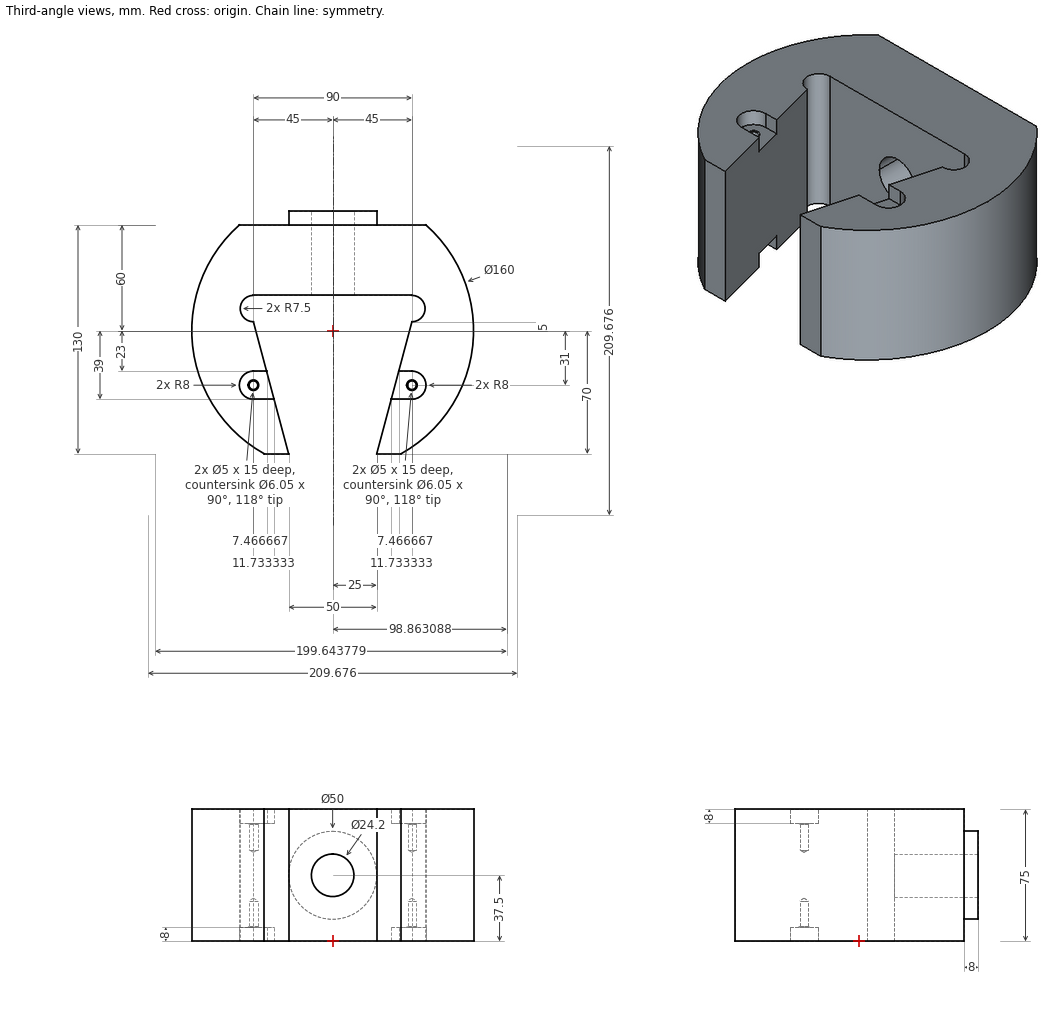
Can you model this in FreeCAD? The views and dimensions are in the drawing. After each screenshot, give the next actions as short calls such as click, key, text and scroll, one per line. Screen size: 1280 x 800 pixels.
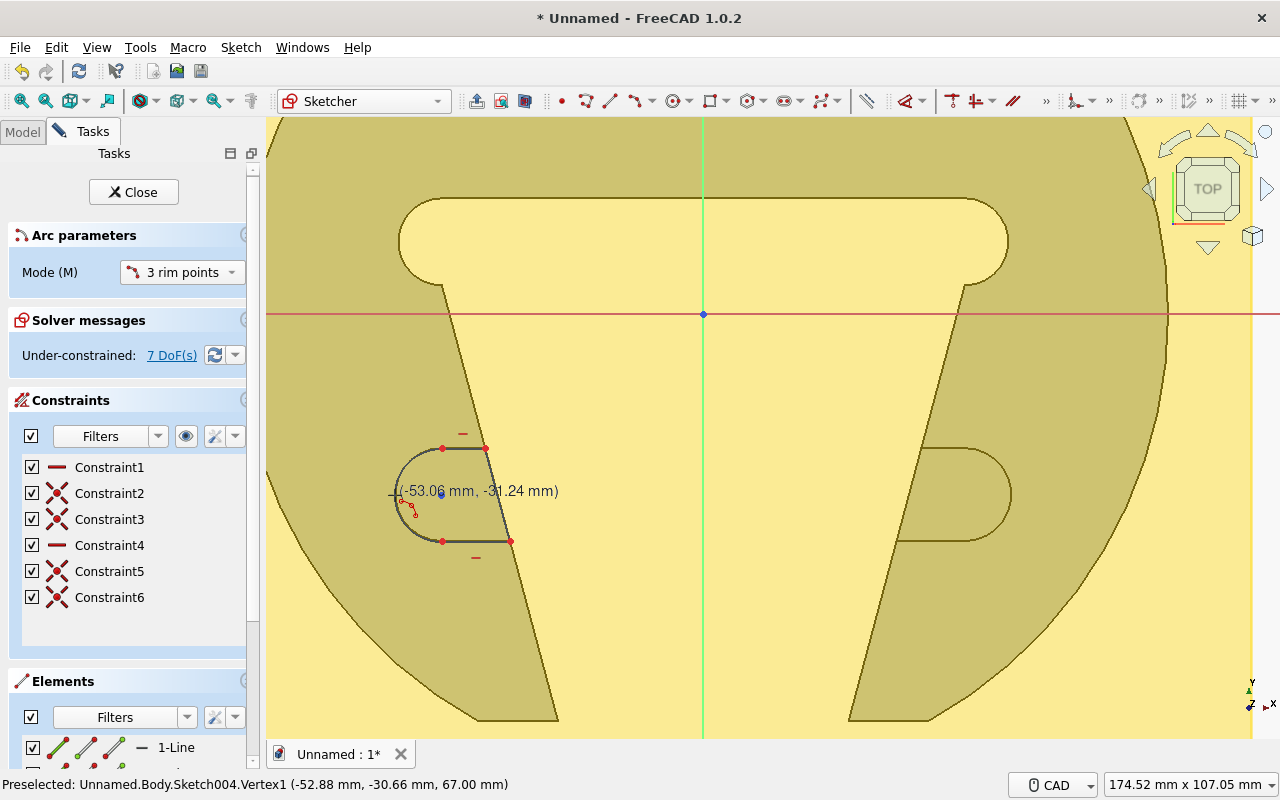
key(g)
key(m)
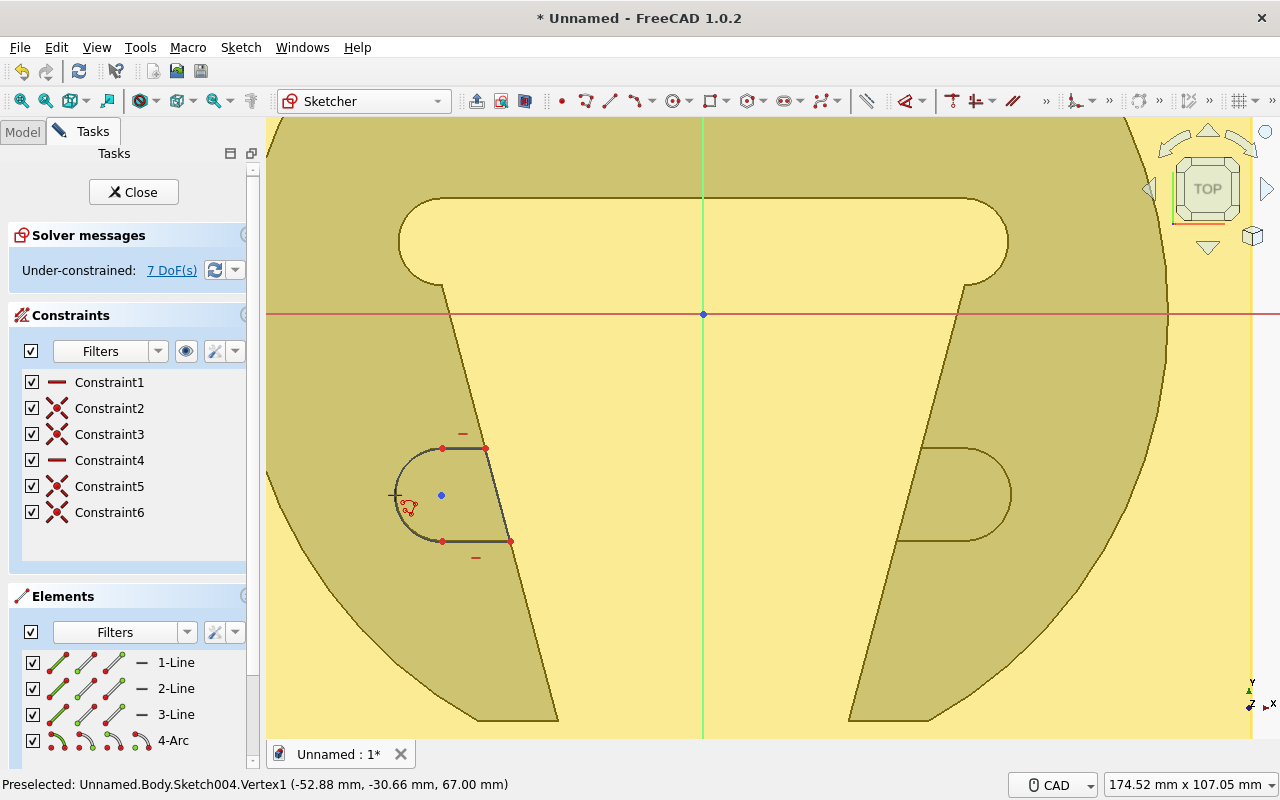
click(965, 541)
click(897, 541)
click(921, 448)
click(965, 448)
right_click(965, 448)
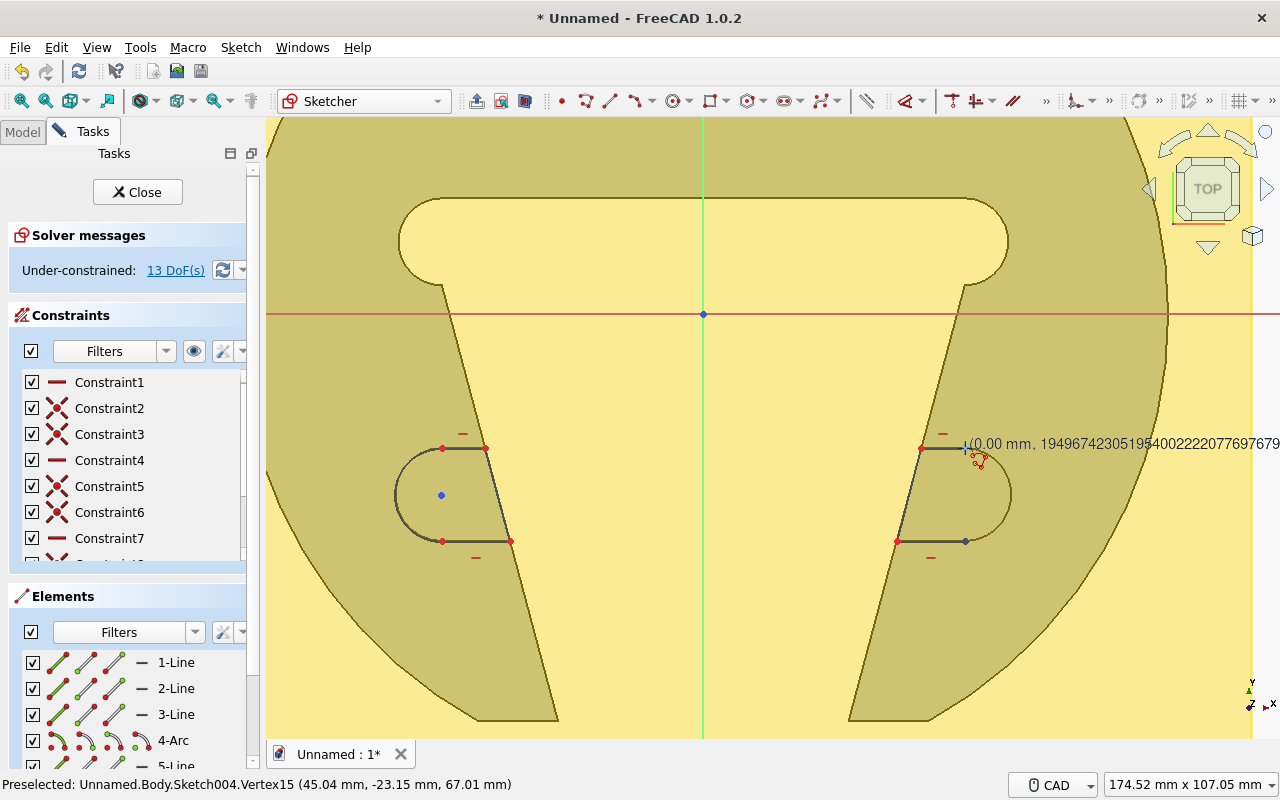
key(g)
key(3)
key(a)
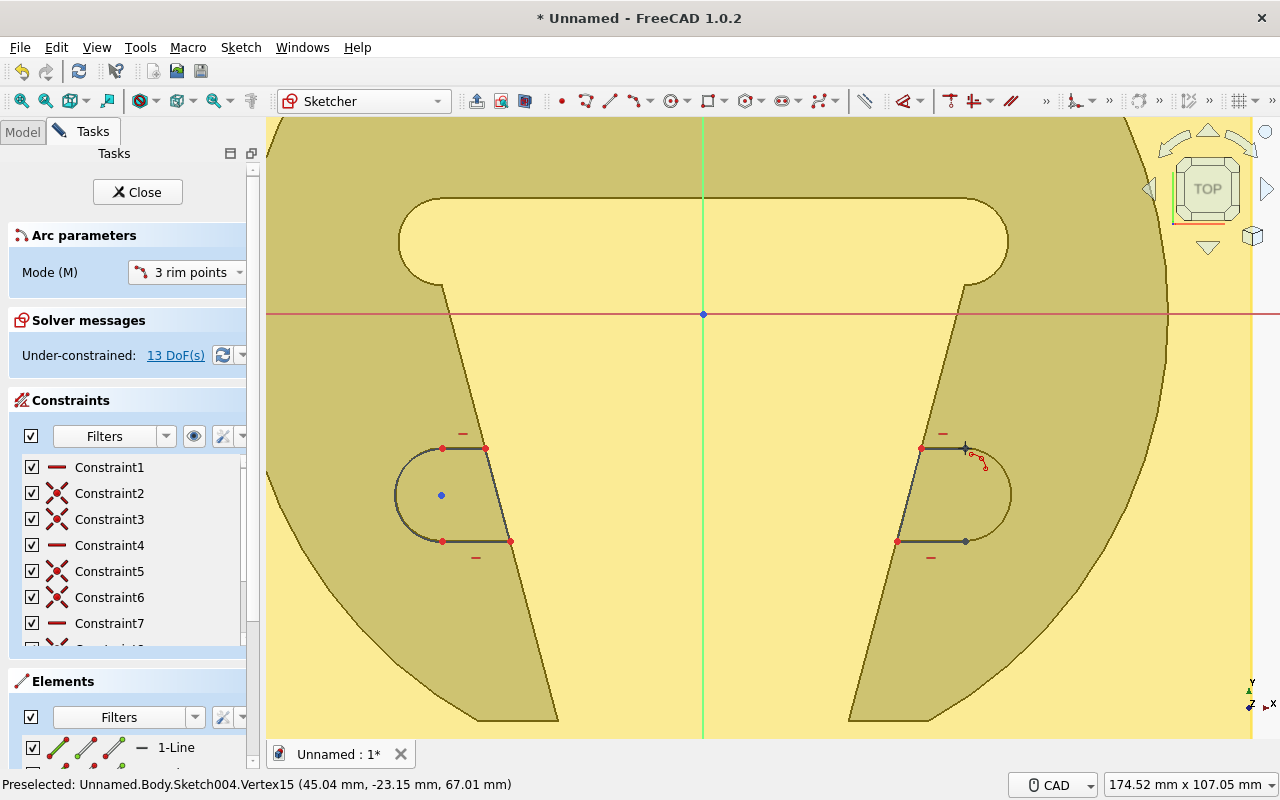
click(965, 449)
click(965, 542)
click(1011, 495)
key(Escape)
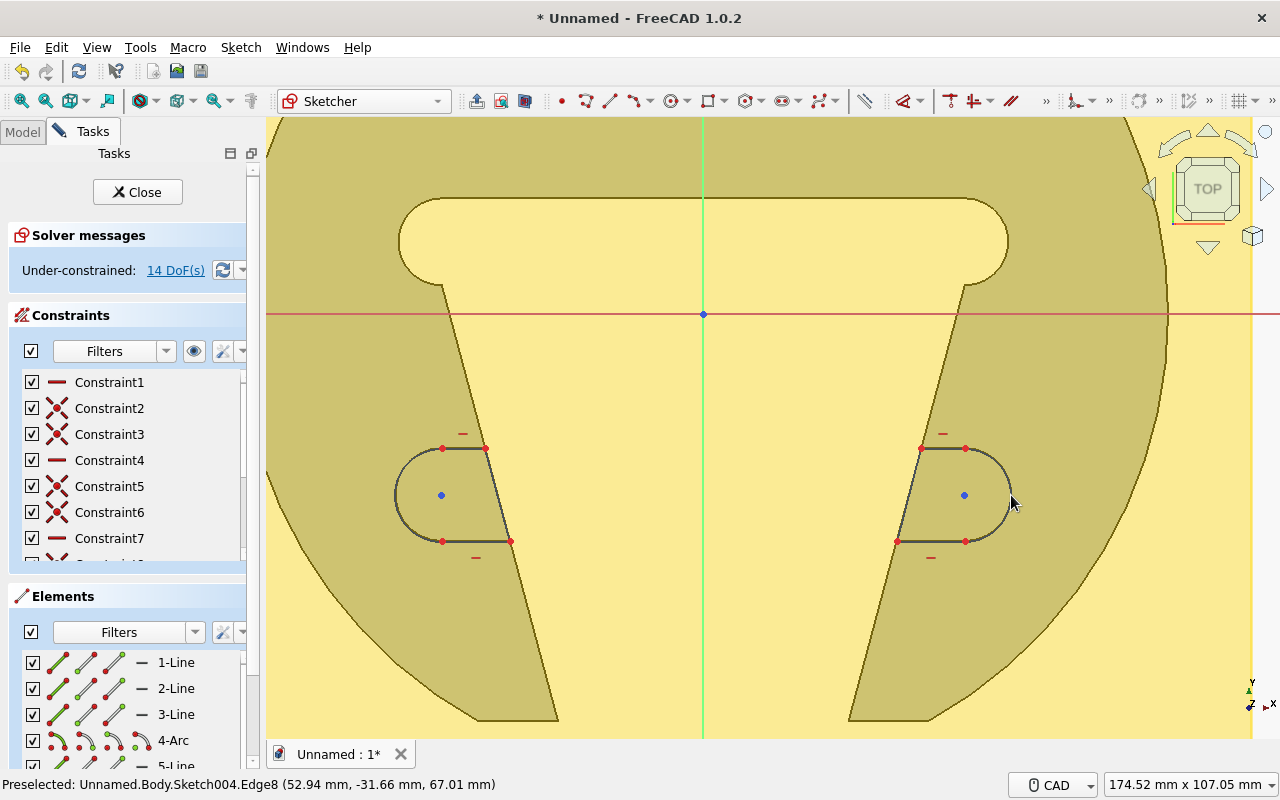
click(455, 449)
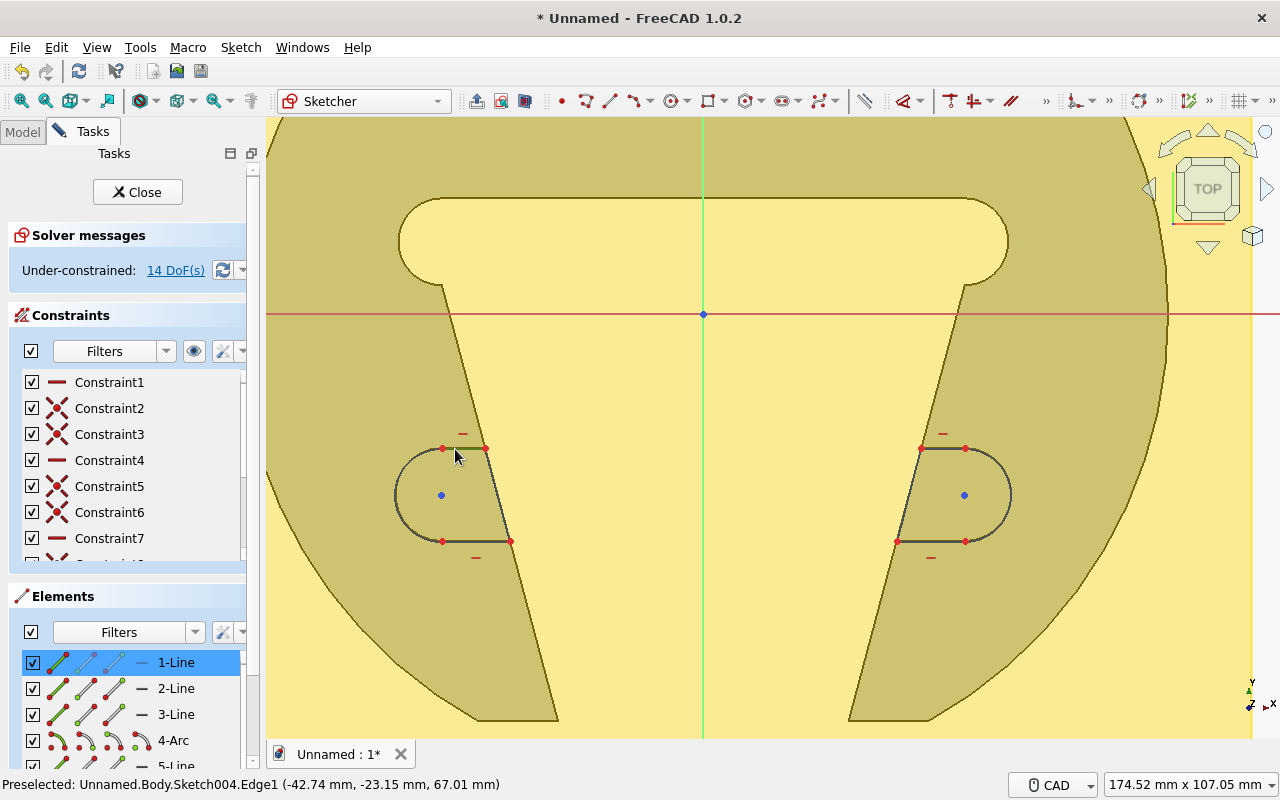
click(404, 468)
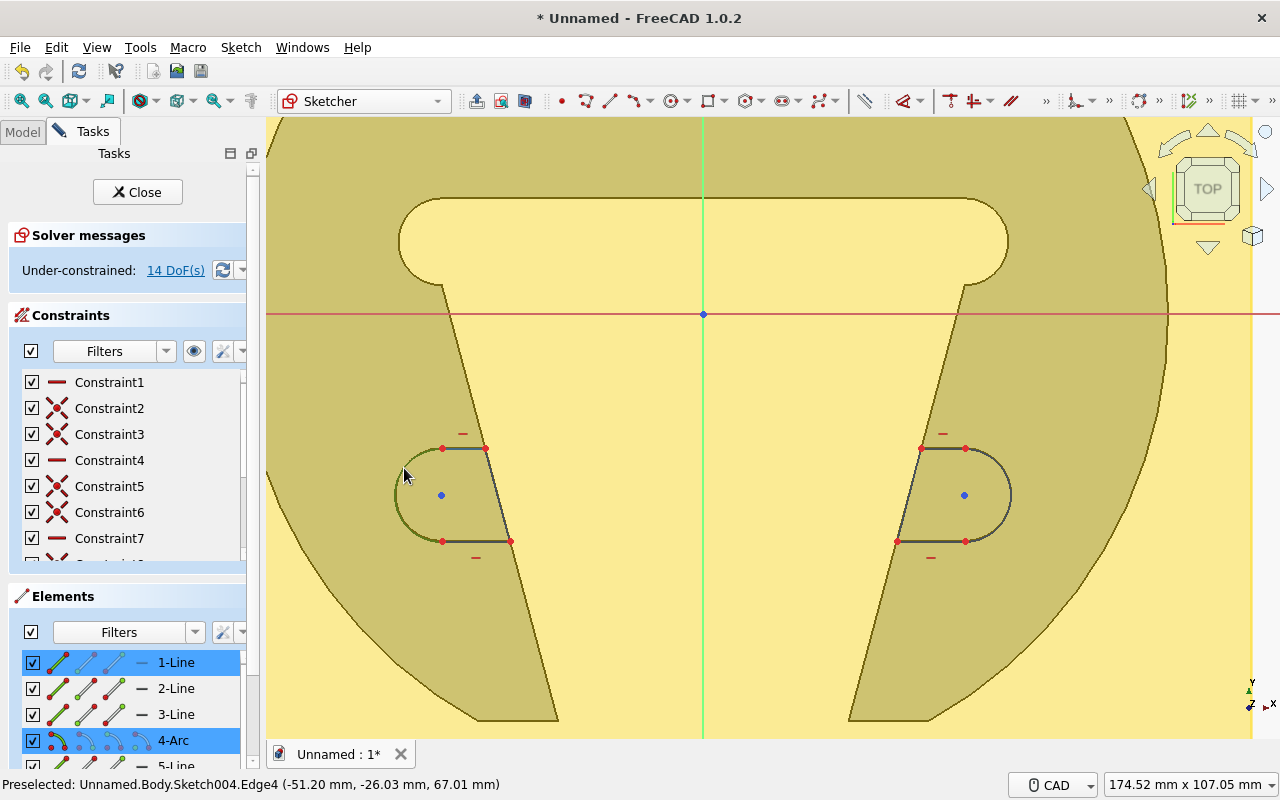
key(t)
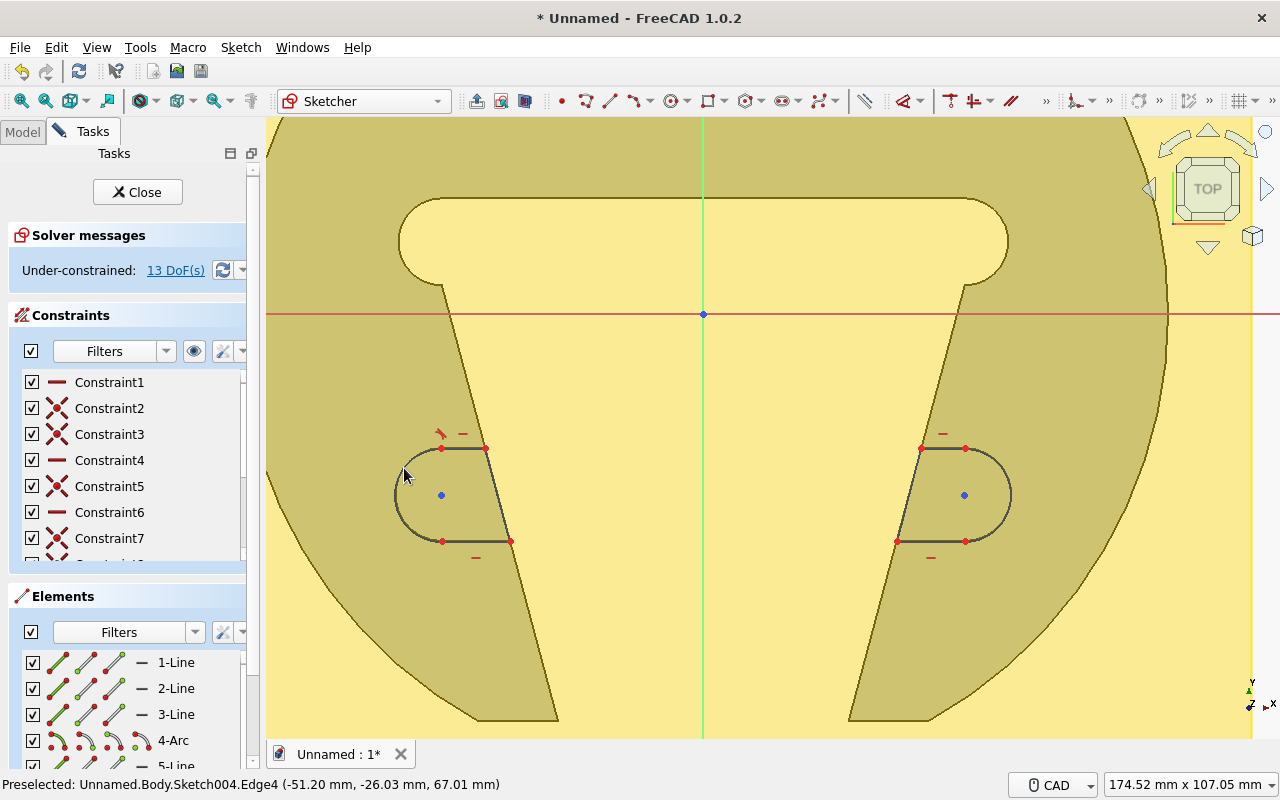
click(490, 542)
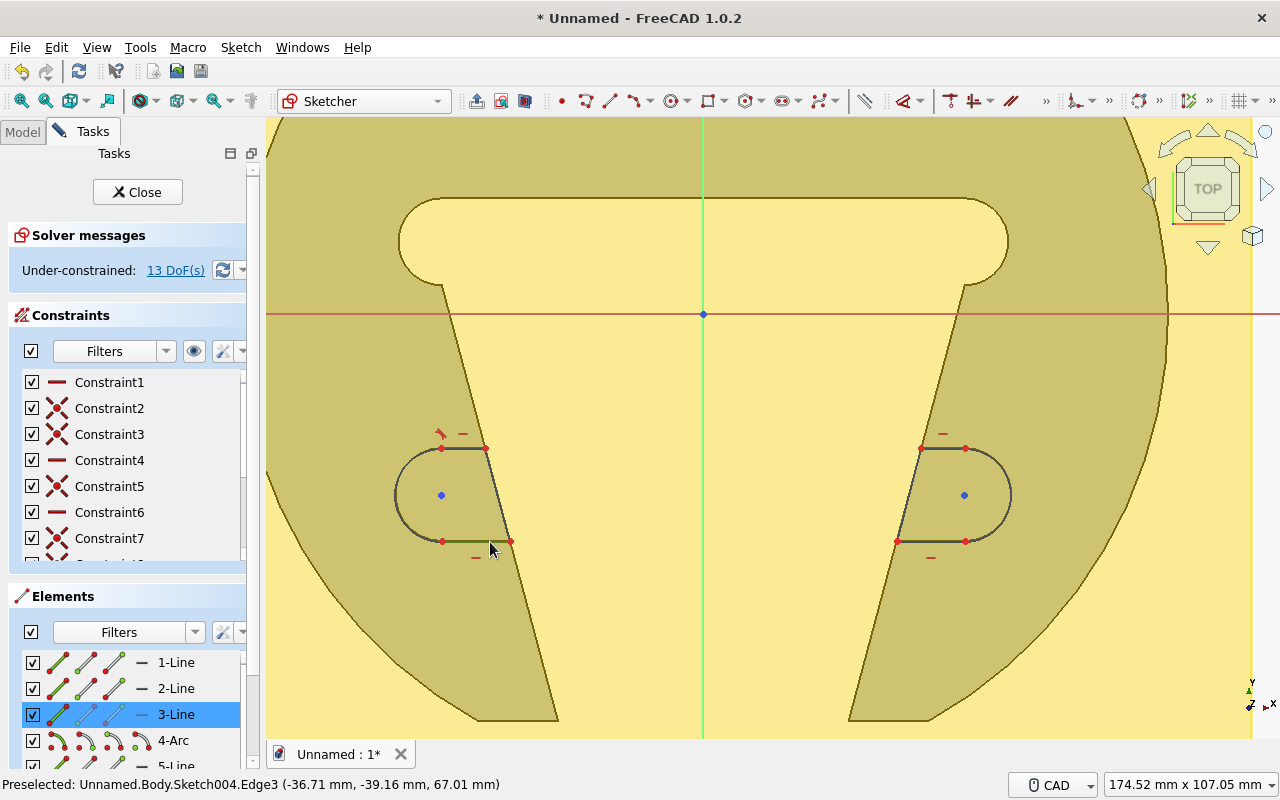
click(404, 468)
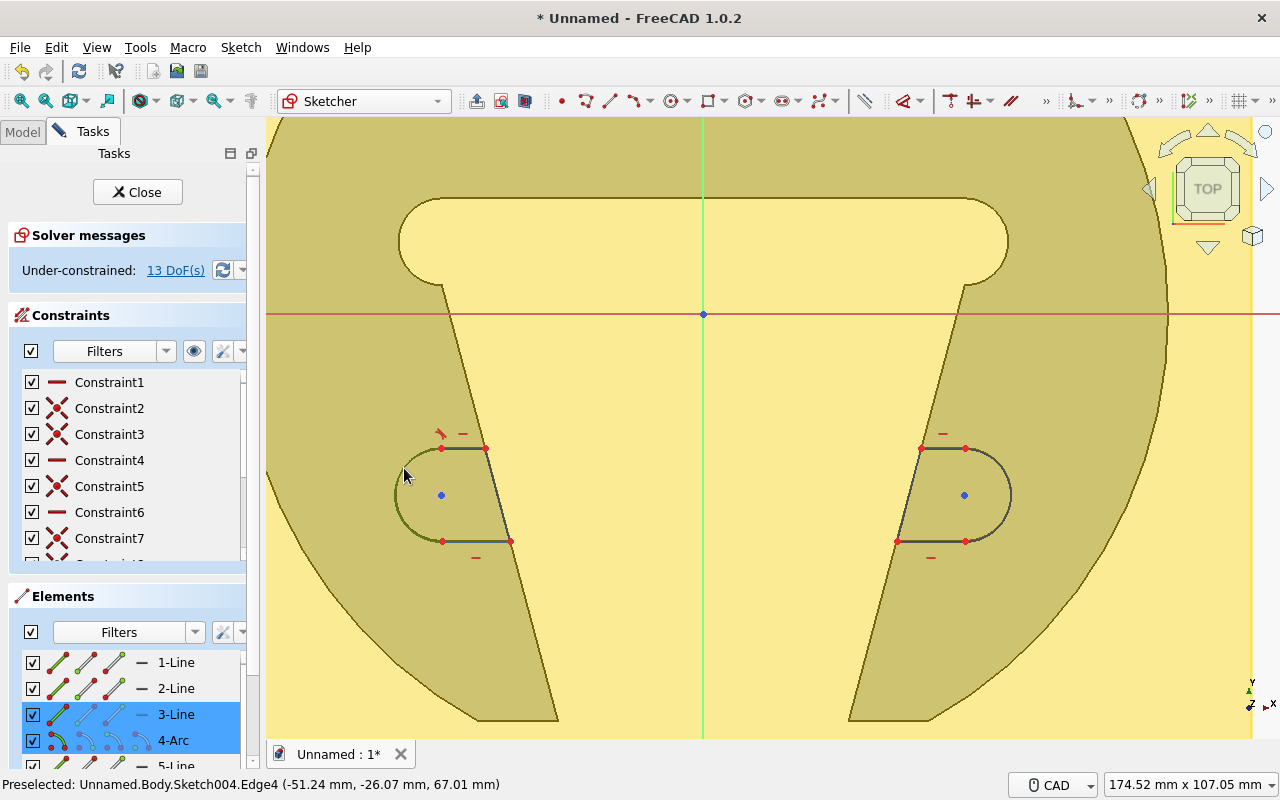
key(t)